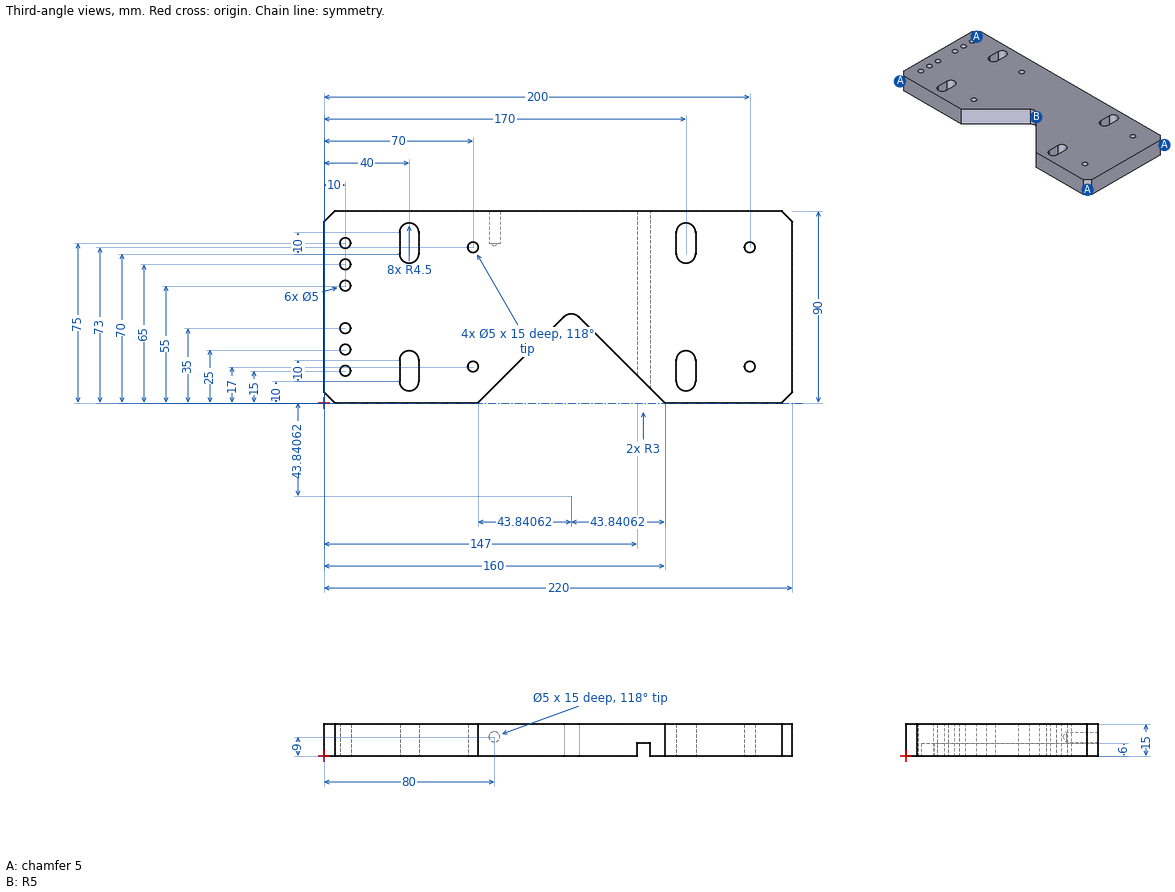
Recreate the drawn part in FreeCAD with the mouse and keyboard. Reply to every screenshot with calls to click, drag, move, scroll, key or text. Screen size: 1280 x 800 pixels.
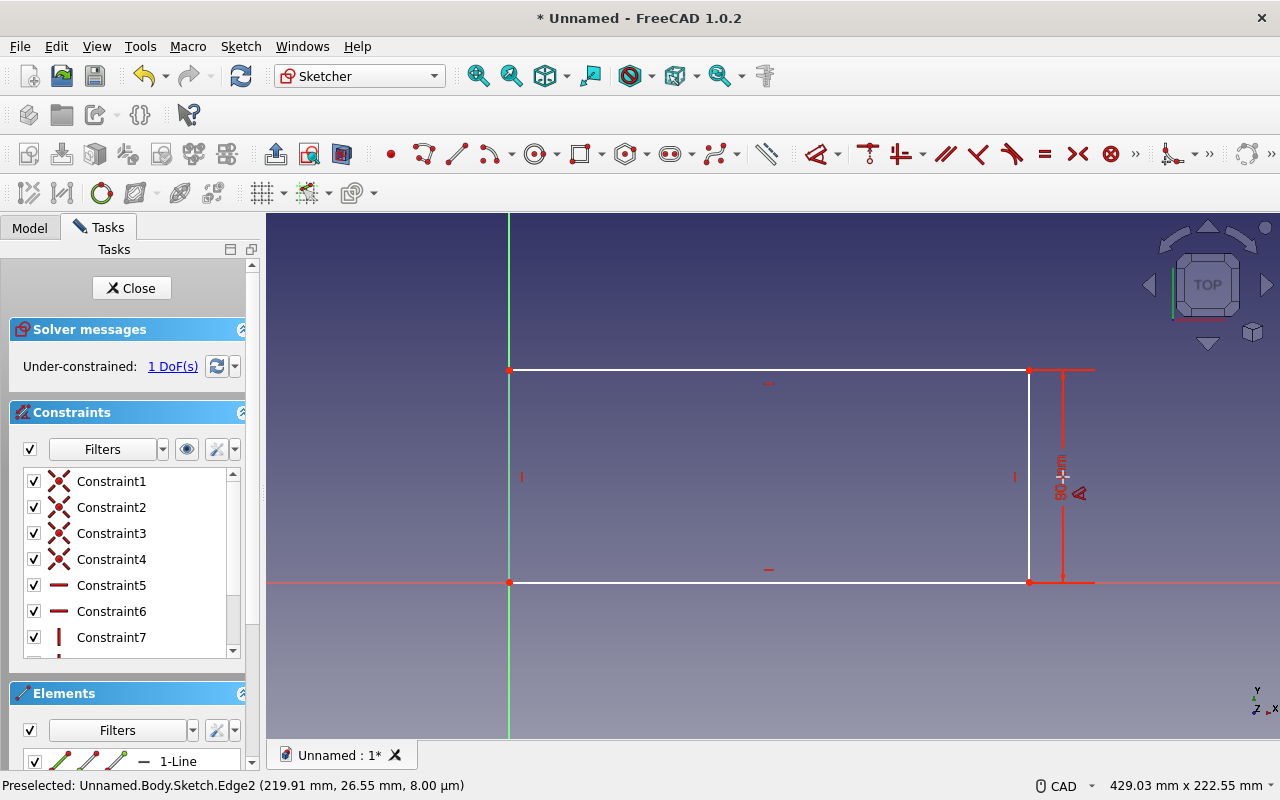
click(665, 583)
click(769, 617)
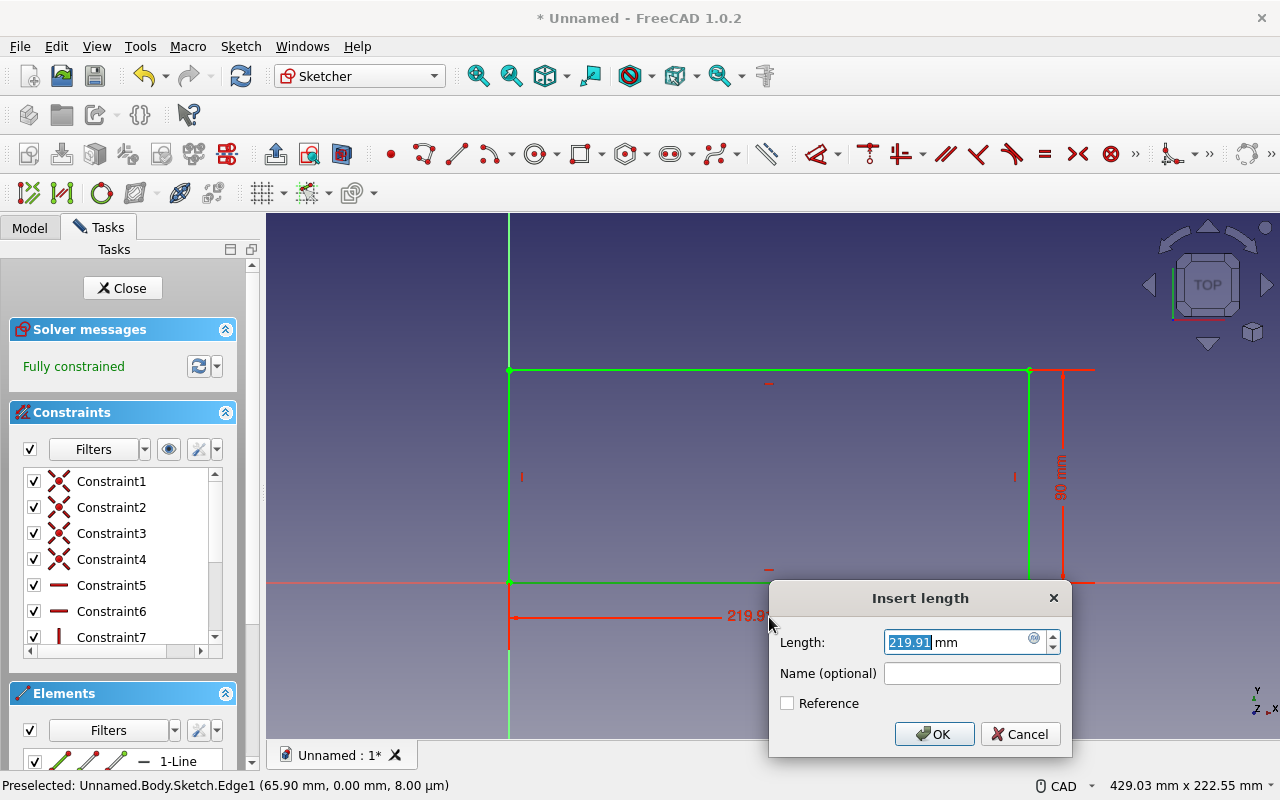
text(220)
key(Return)
key(Escape)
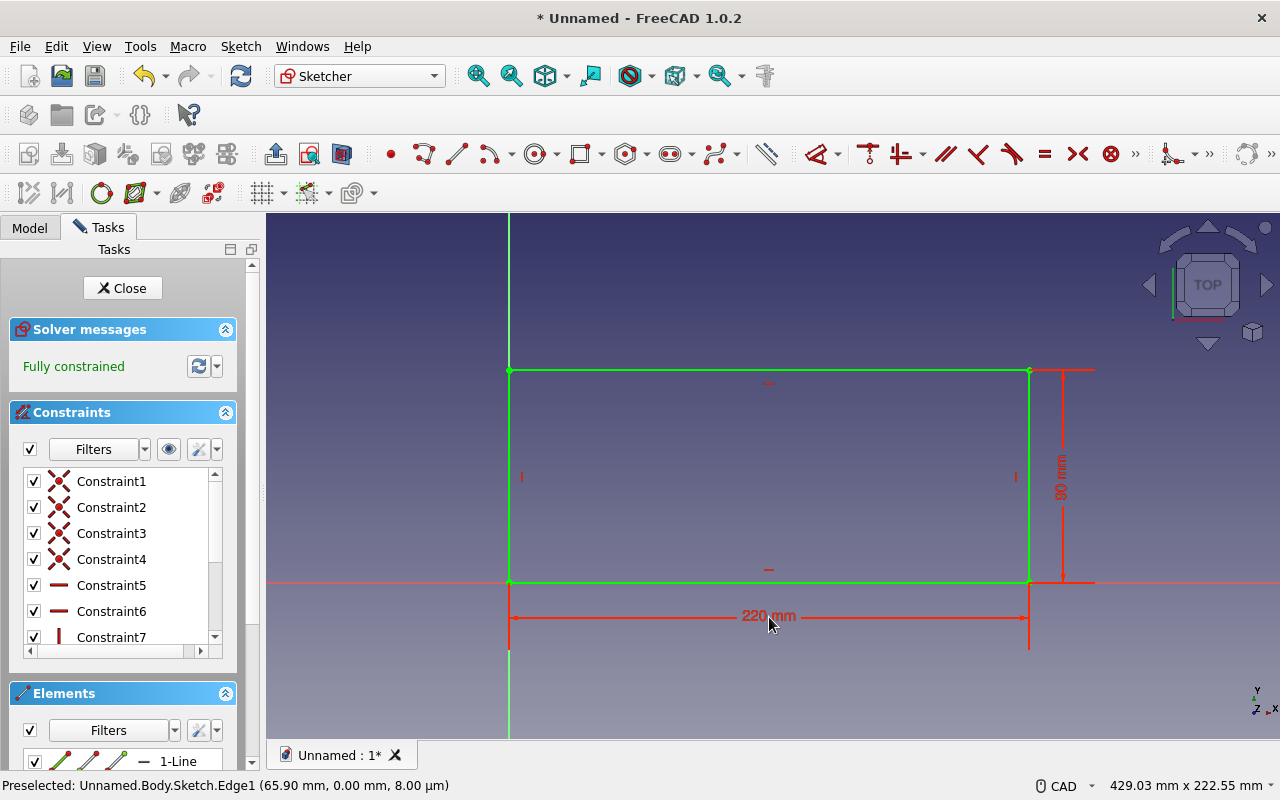
click(123, 288)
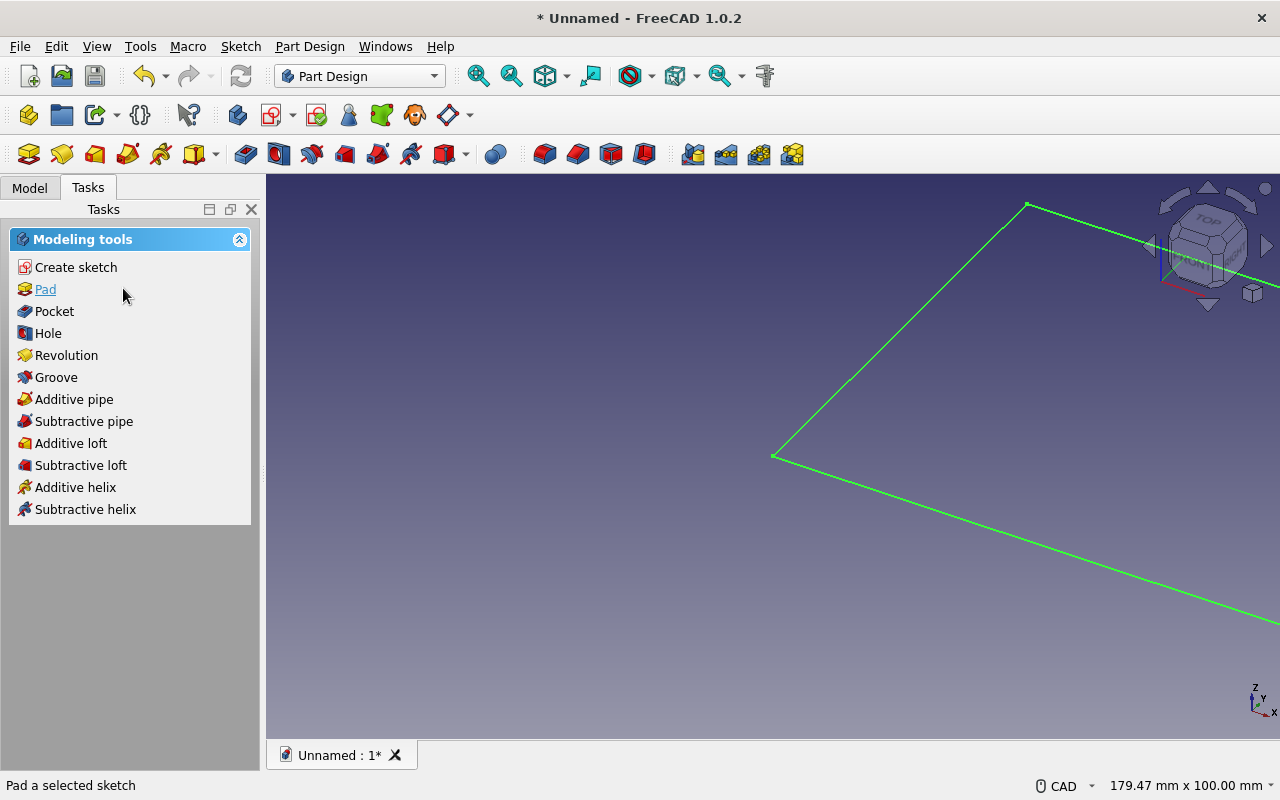
click(29, 154)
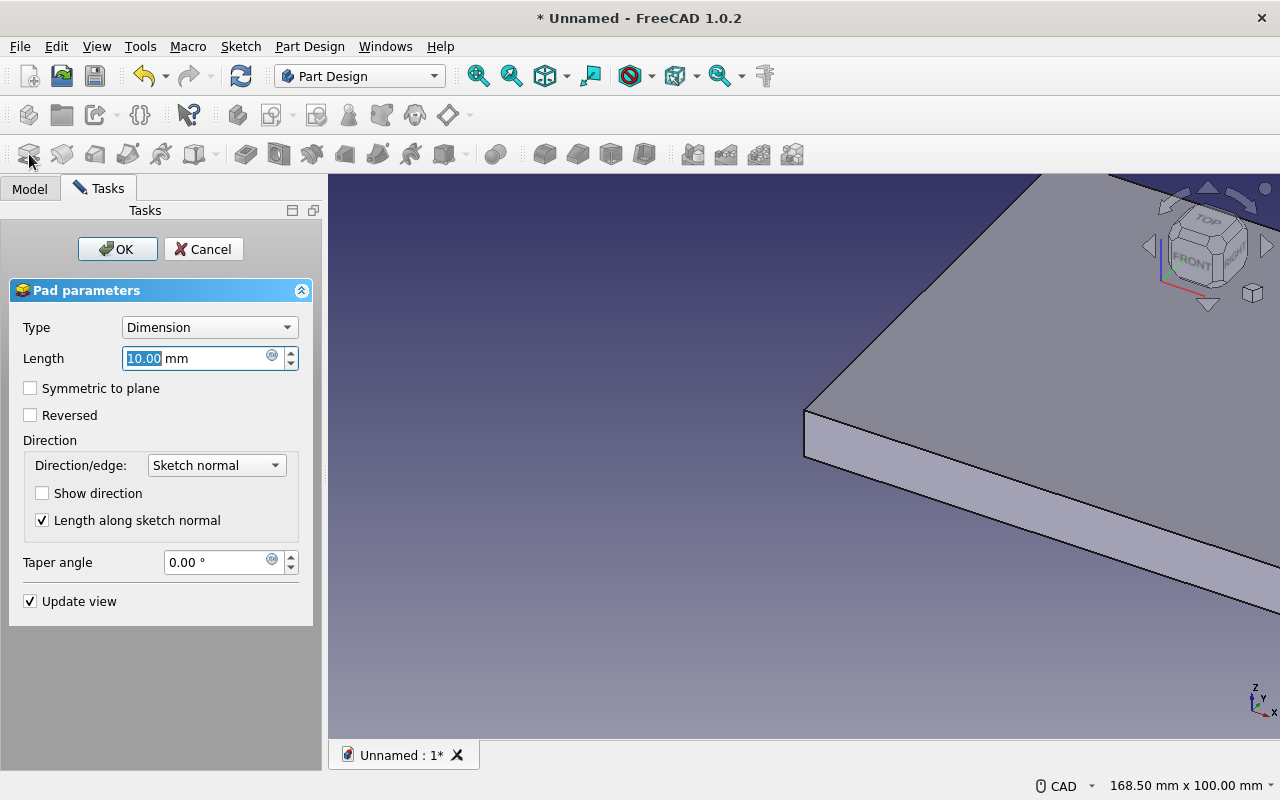
text(15)
key(Tab)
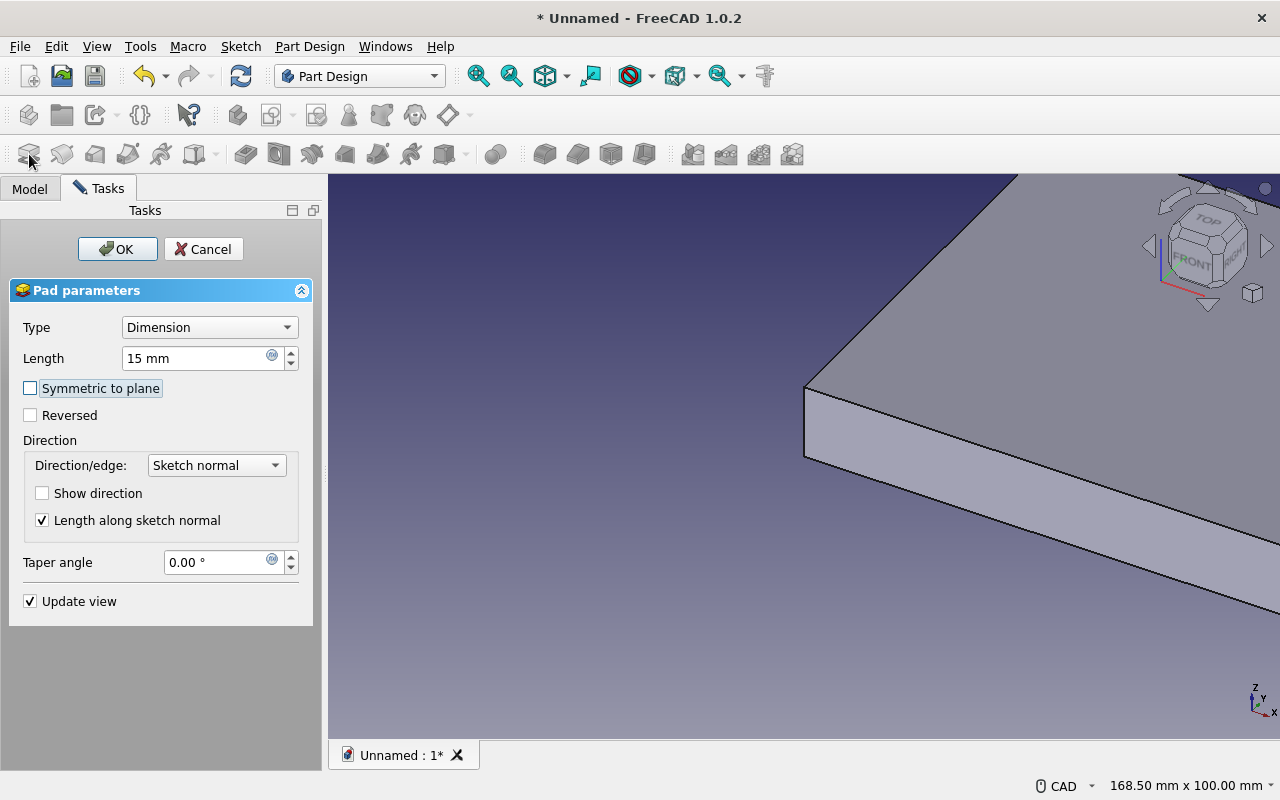
click(118, 249)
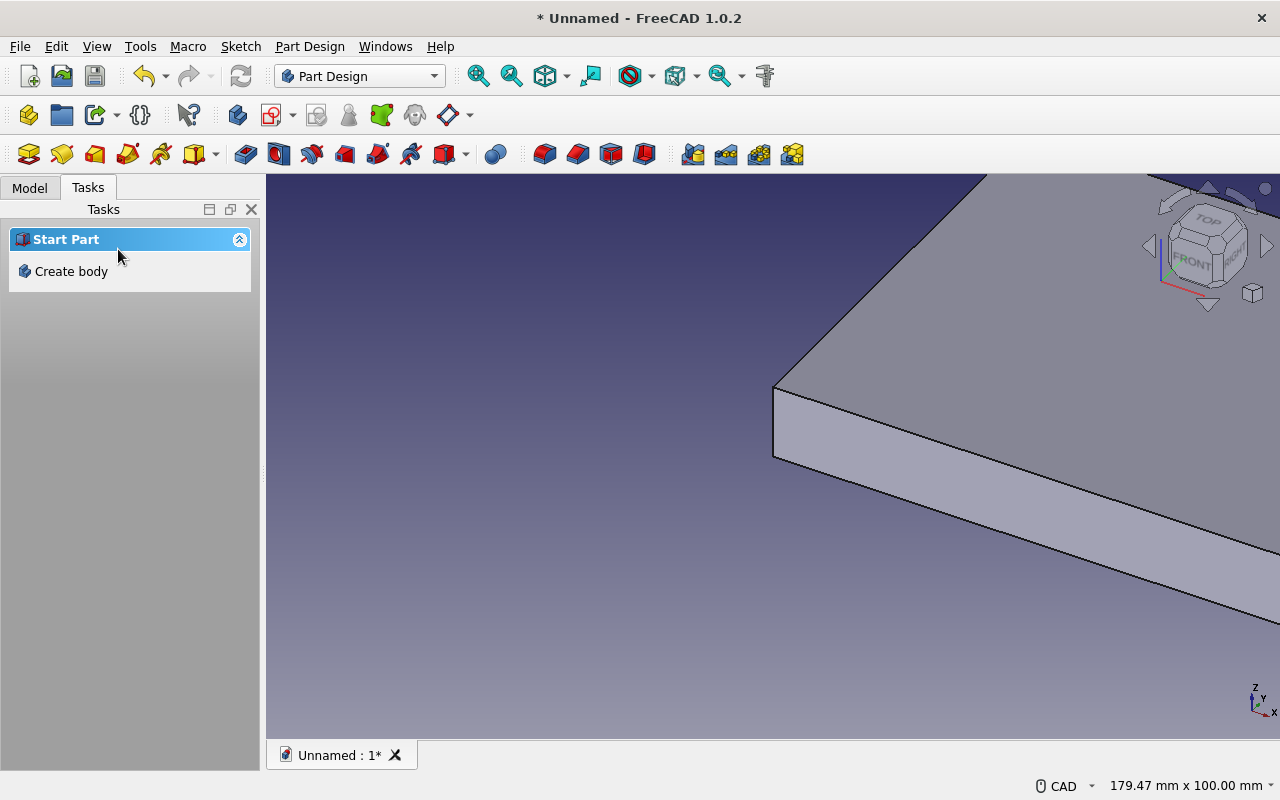
click(479, 76)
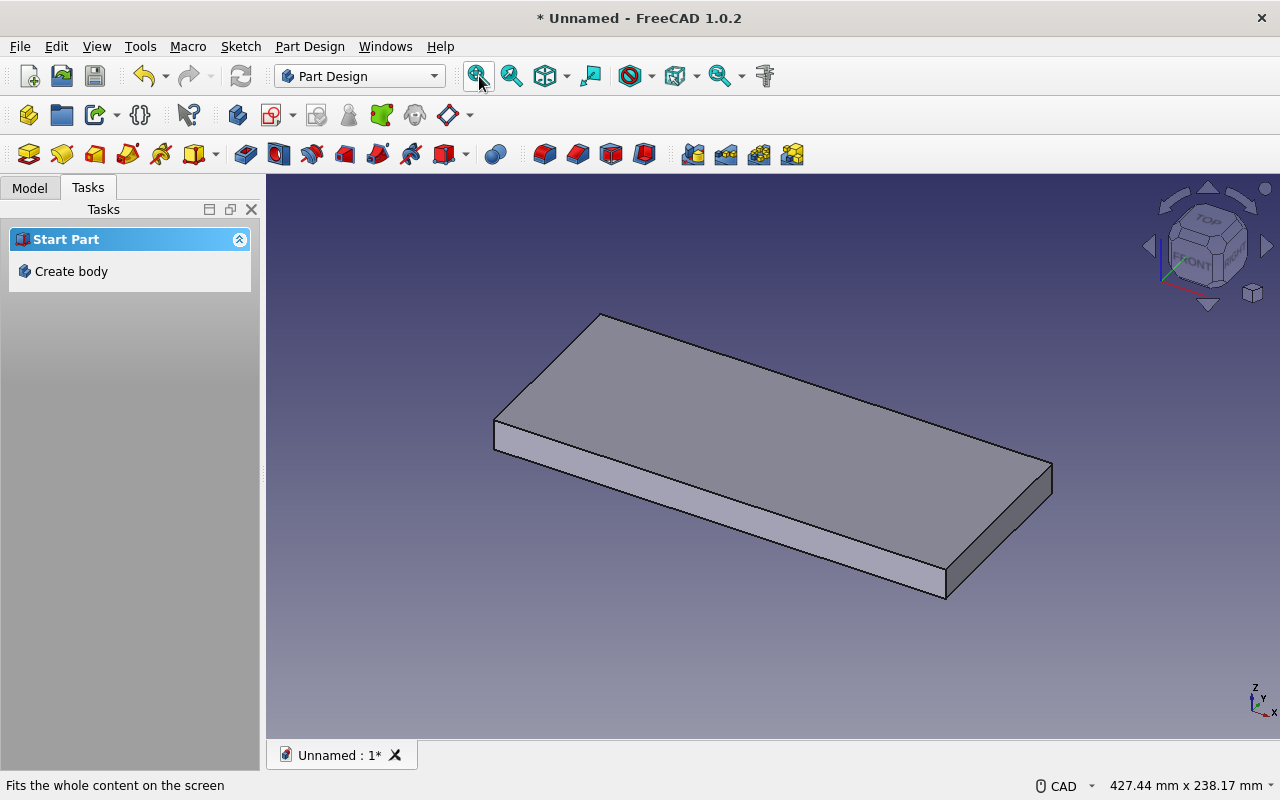
click(902, 484)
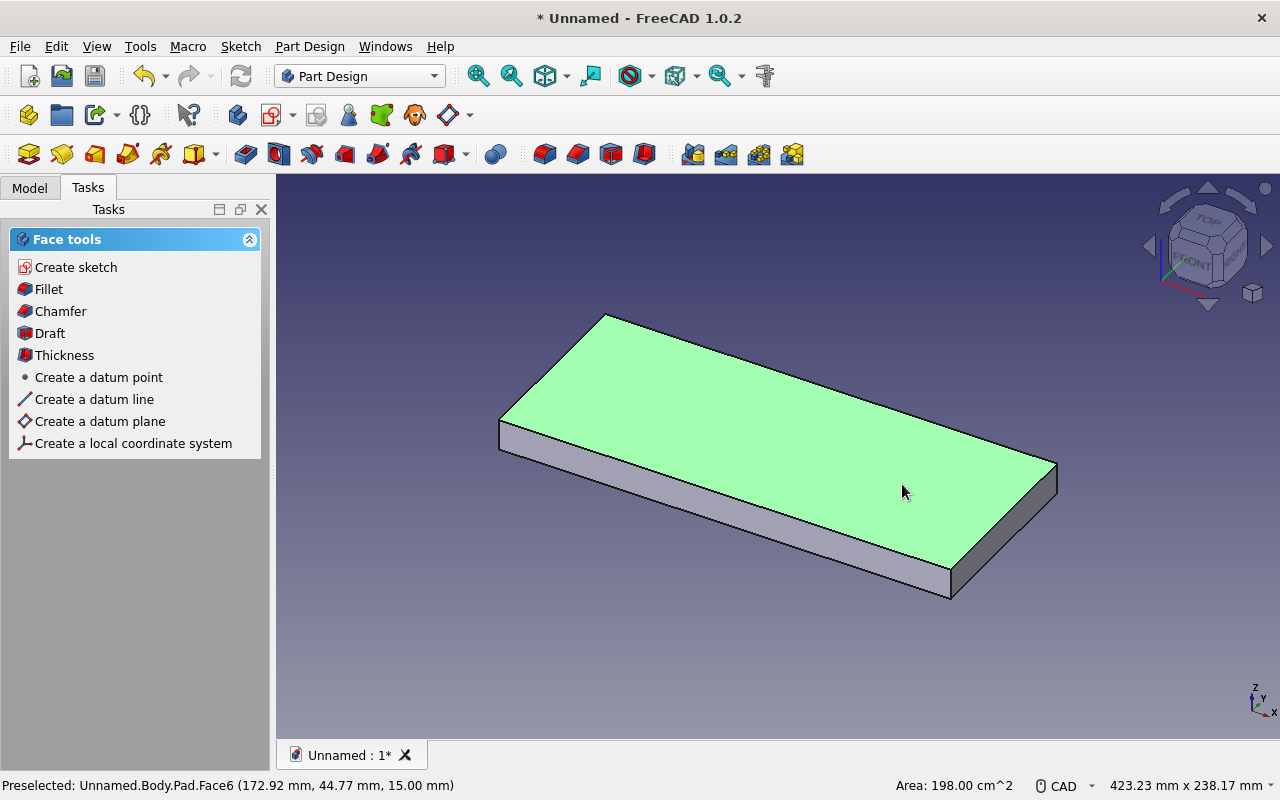
click(270, 116)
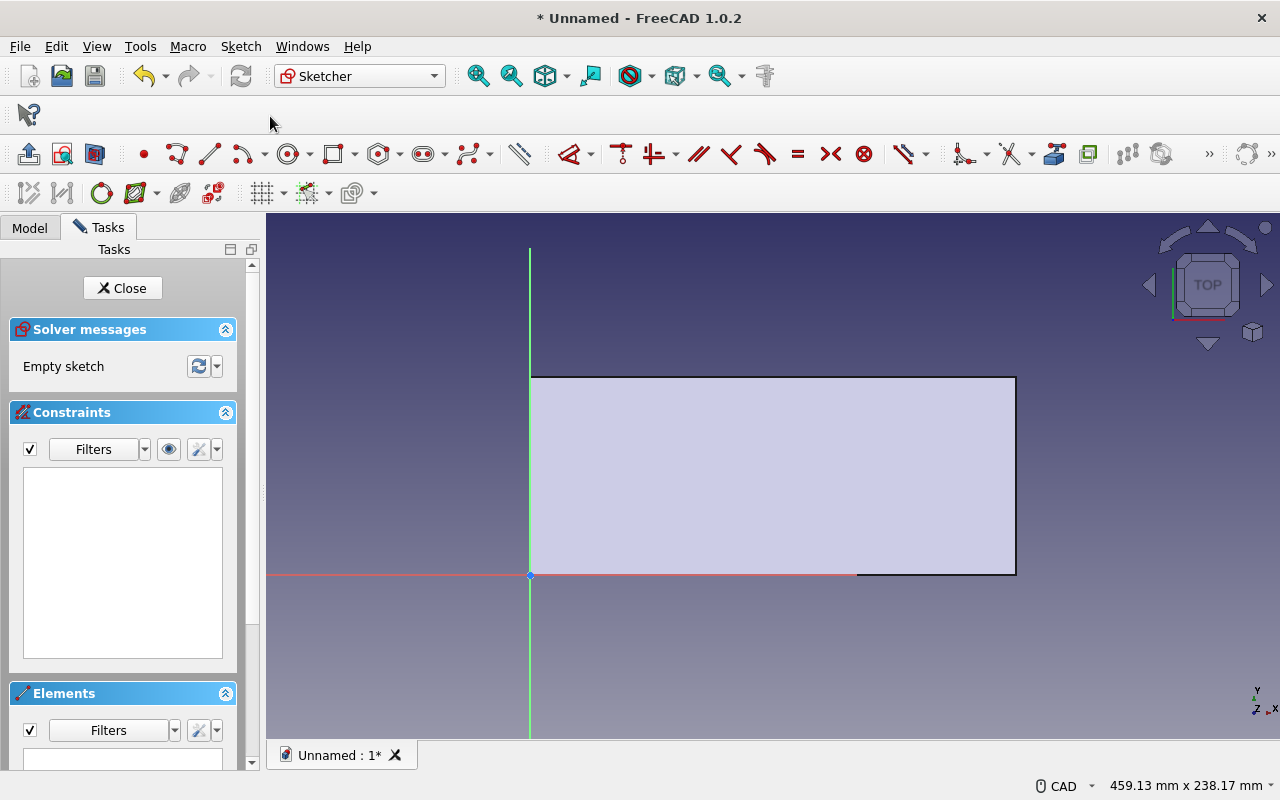
key(g)
key(c)